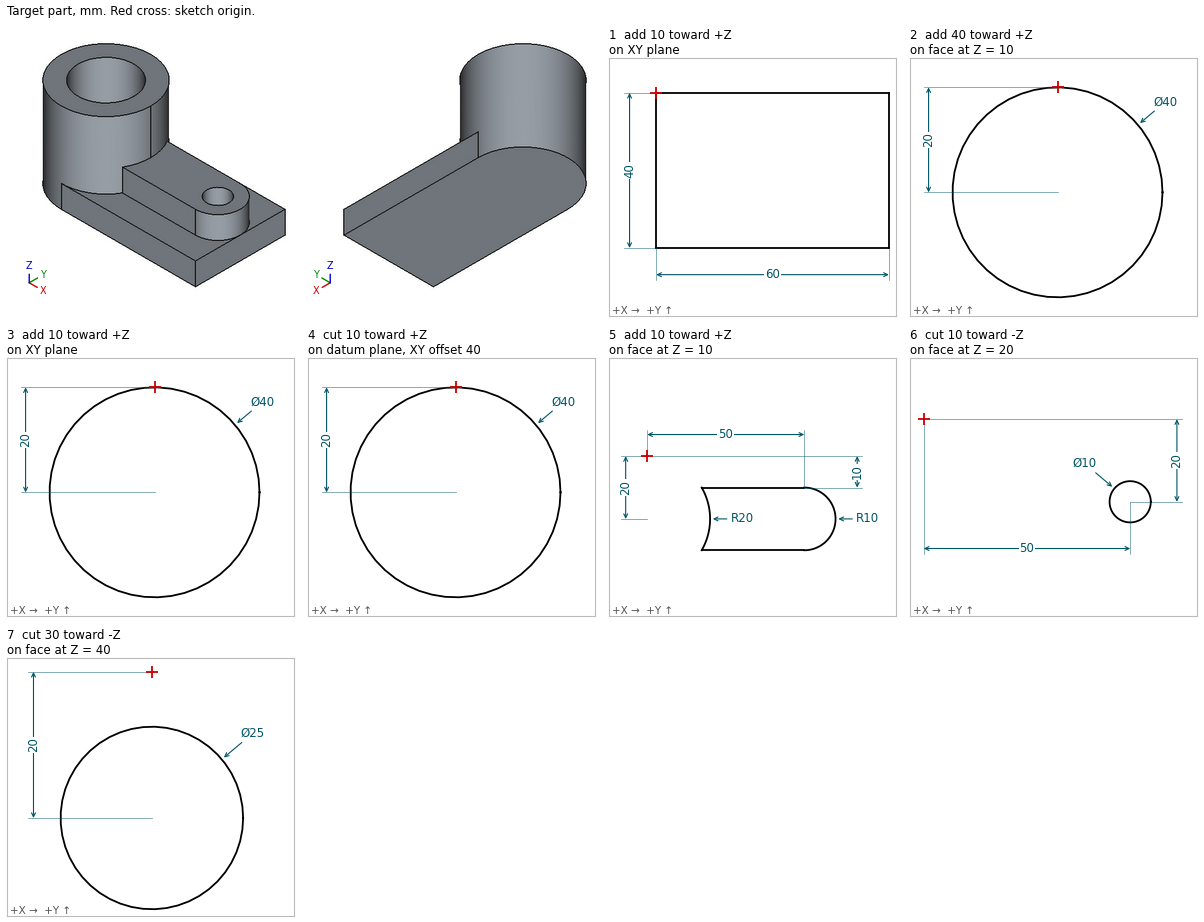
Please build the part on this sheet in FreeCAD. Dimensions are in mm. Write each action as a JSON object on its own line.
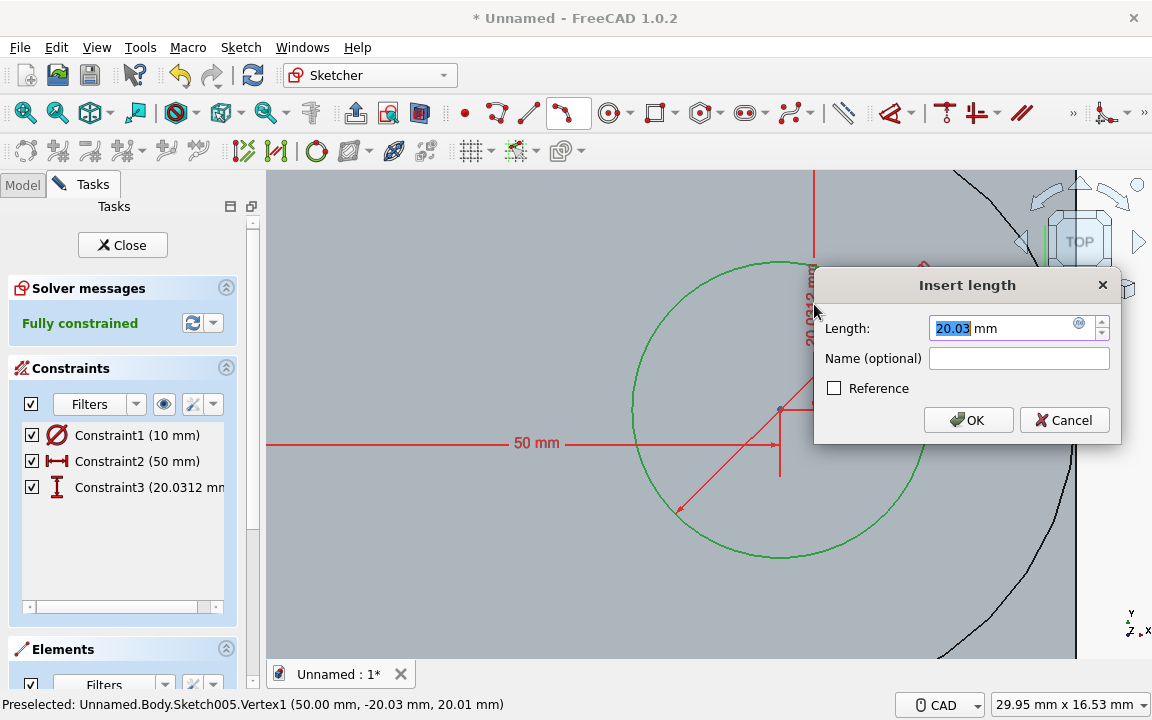
{"action": "type", "text": "20"}
{"action": "key", "text": "Return"}
{"action": "key", "text": "Escape"}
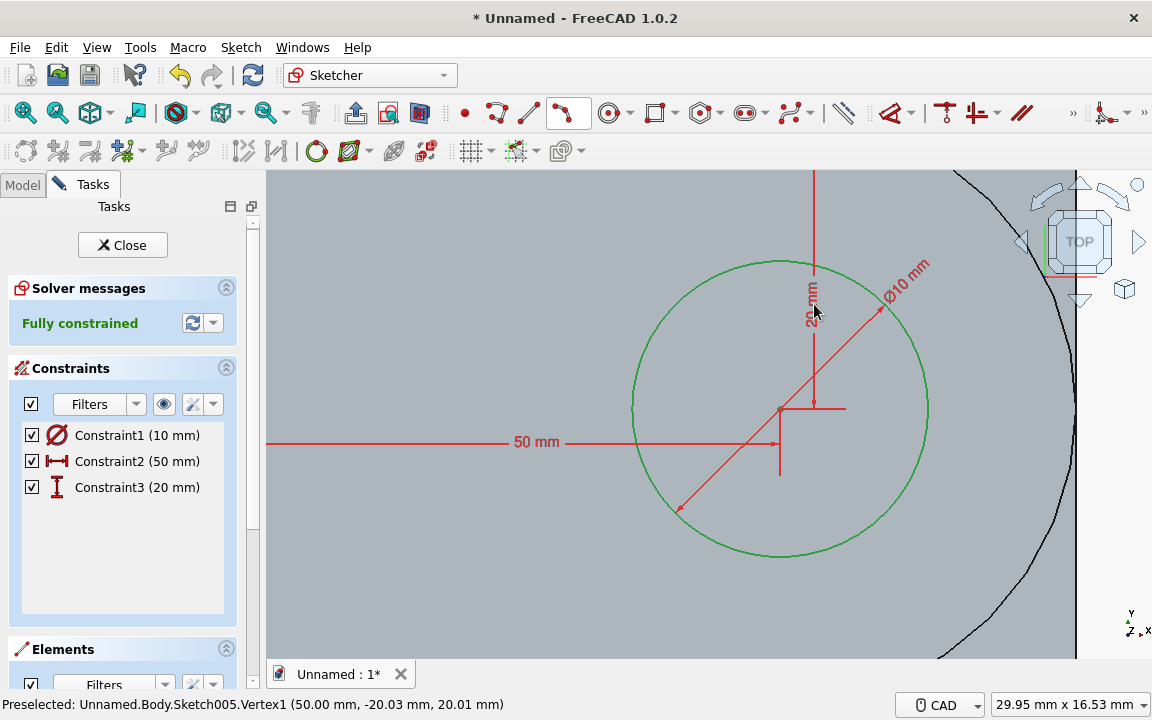
{"action": "left_click", "coordinate": [123, 245]}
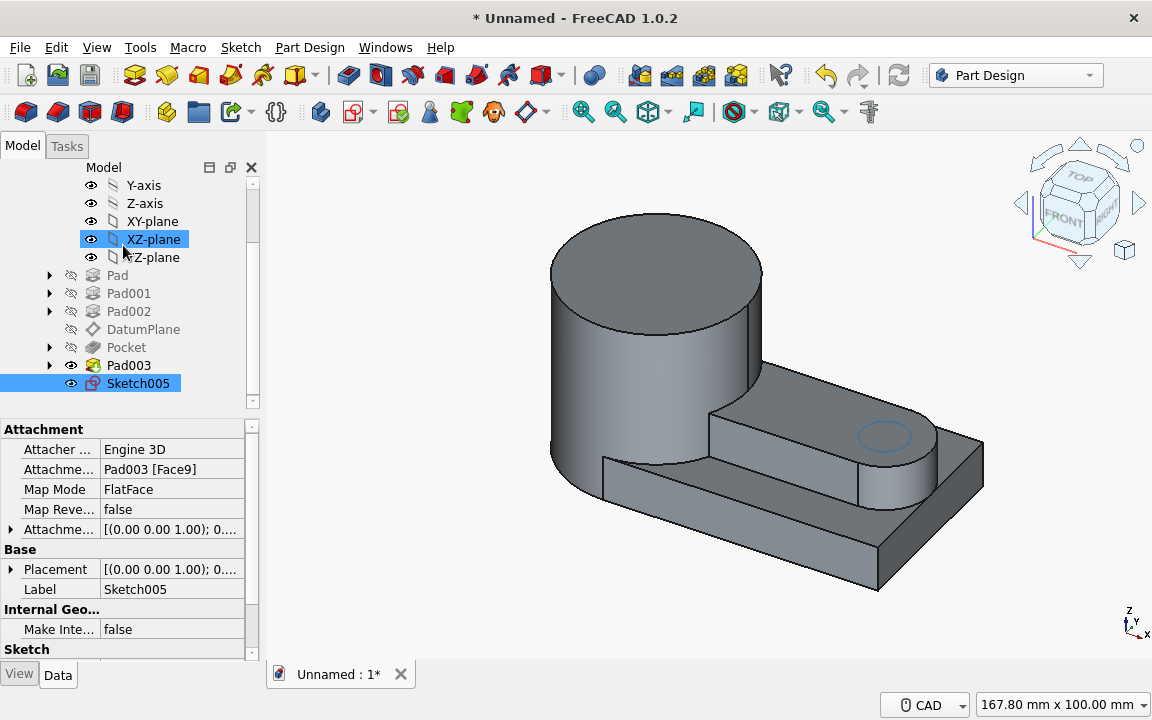
{"action": "left_click", "coordinate": [350, 76]}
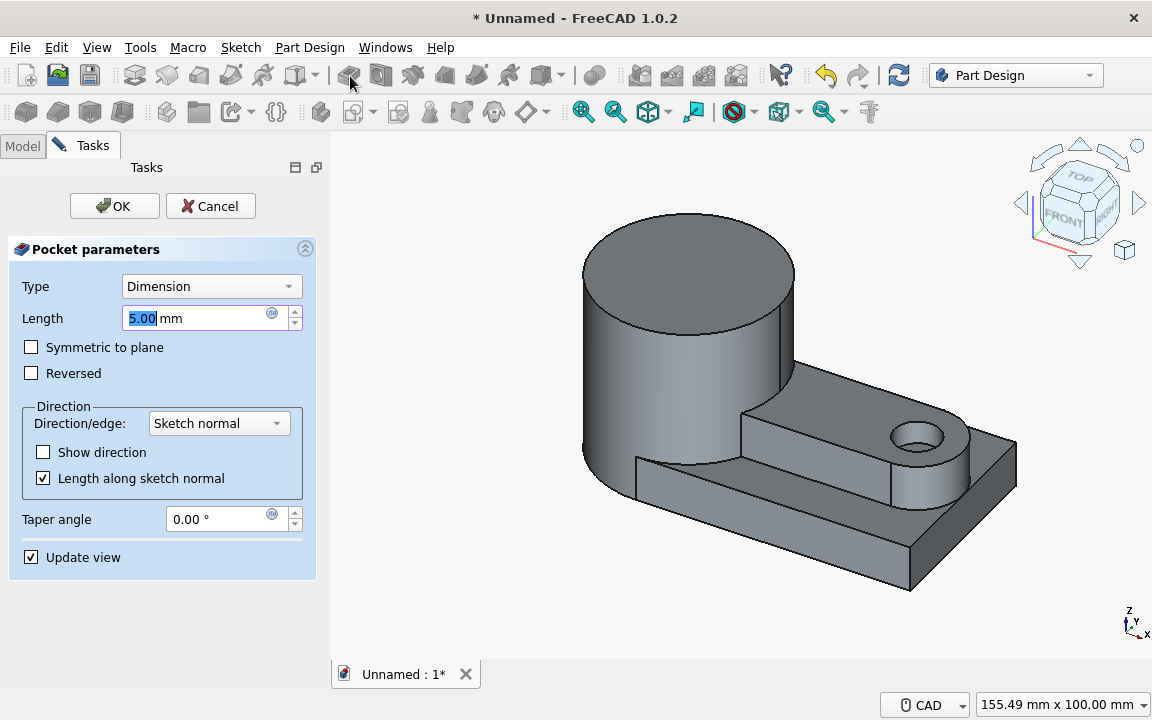
{"action": "type", "text": "10"}
{"action": "key", "text": "Tab"}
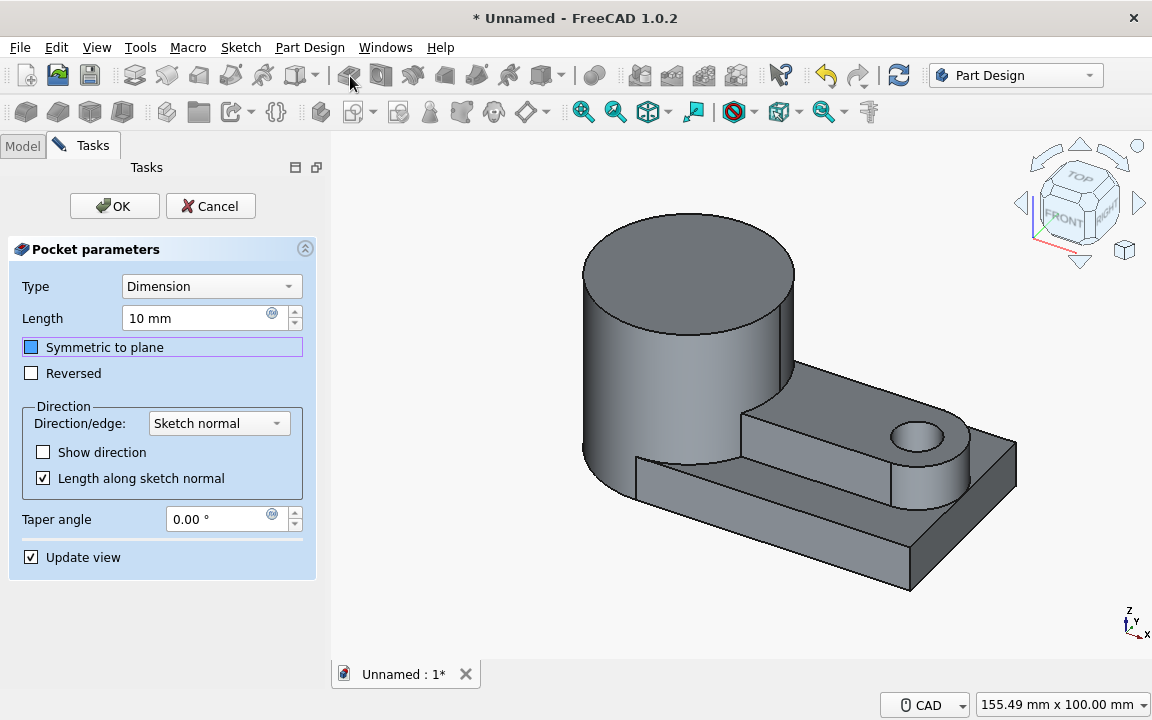
{"action": "left_click", "coordinate": [115, 206]}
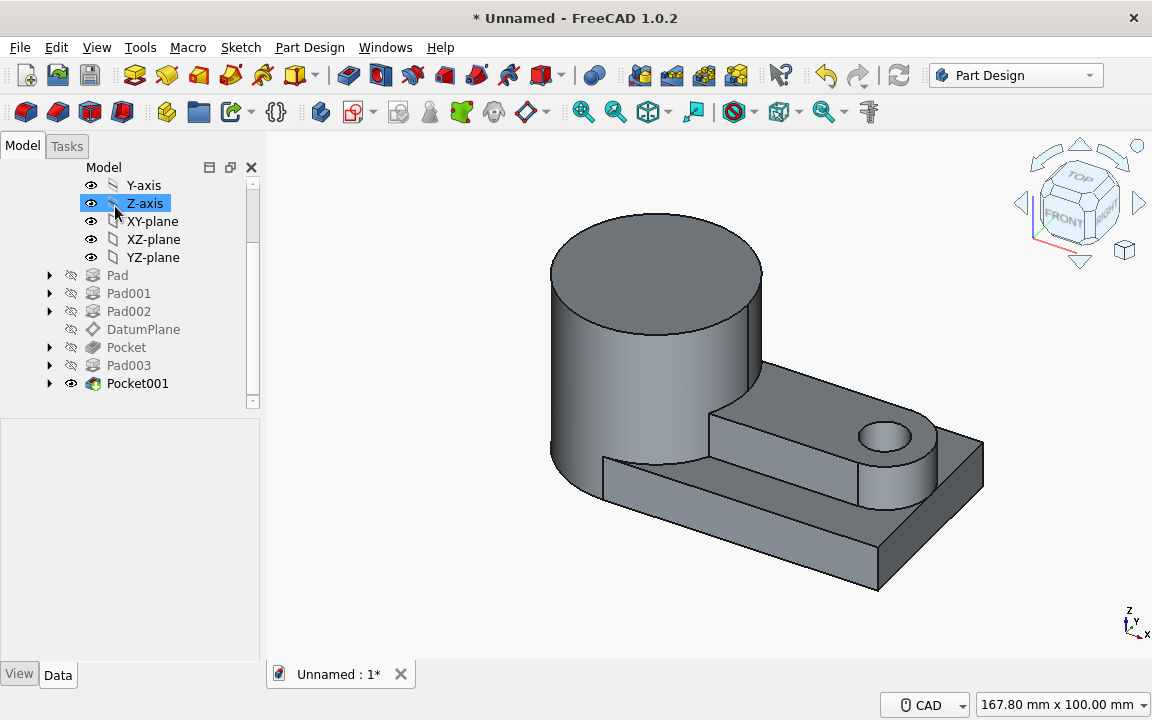
{"action": "left_click", "coordinate": [656, 273]}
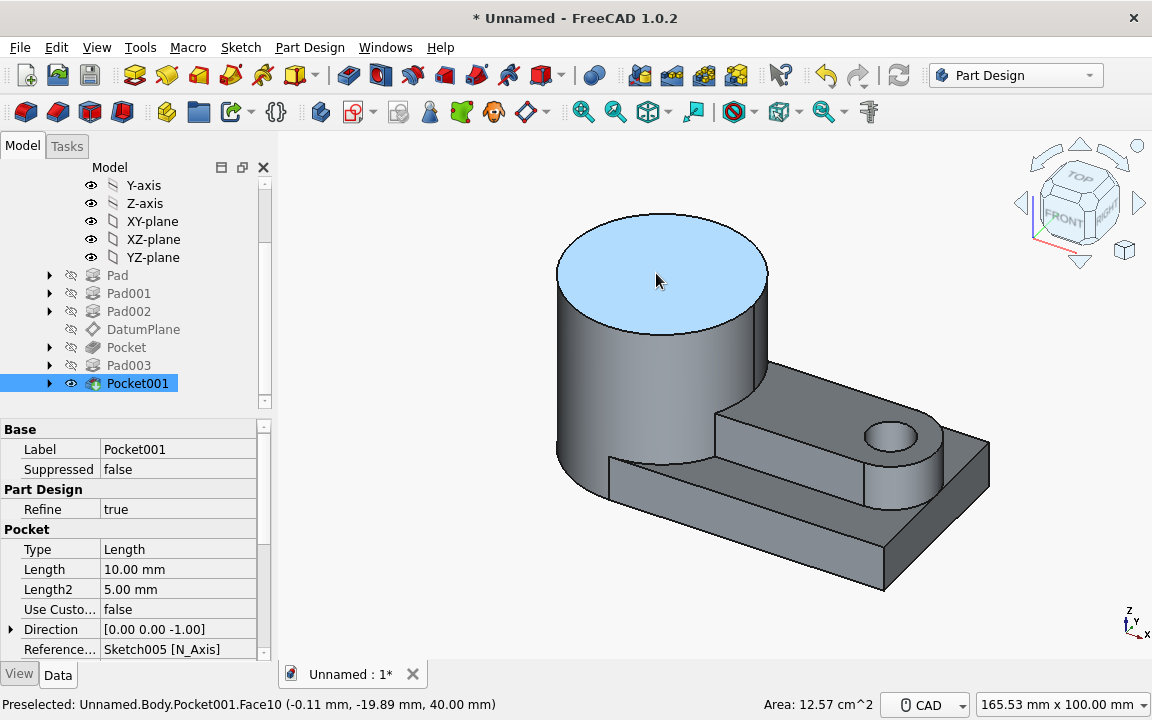
{"action": "left_click", "coordinate": [354, 112]}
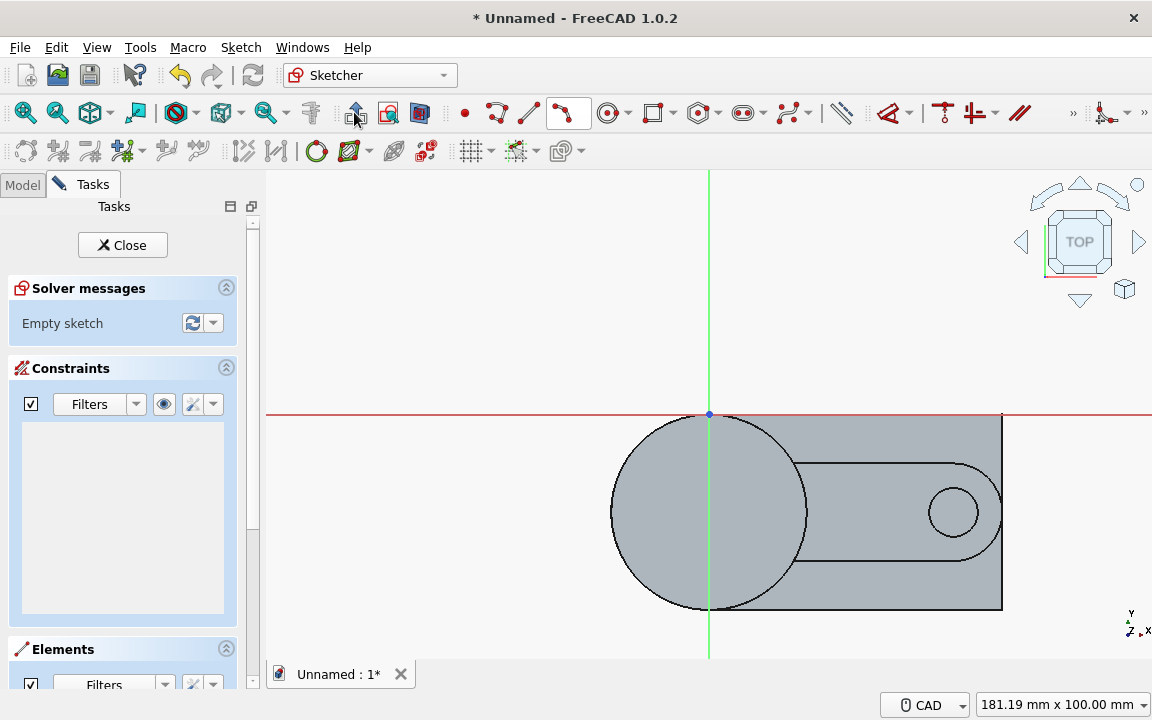
{"action": "scroll", "coordinate": [792, 591], "scroll_direction": "up", "scroll_amount": 3}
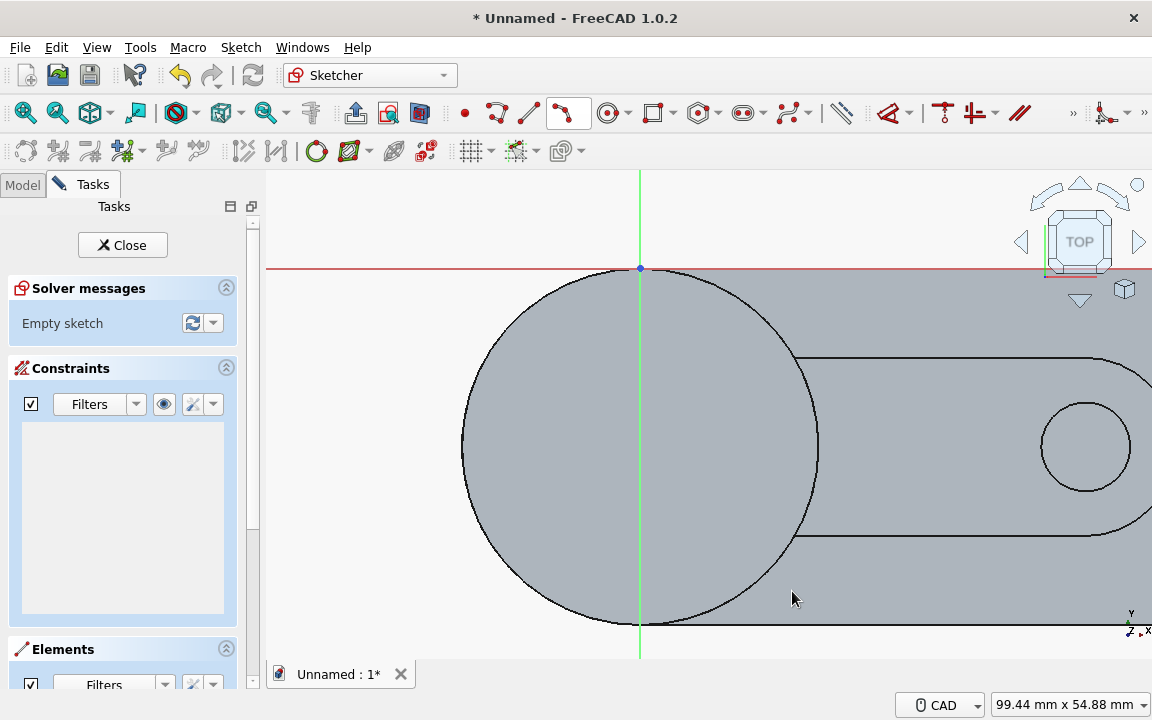
{"action": "left_click", "coordinate": [608, 114]}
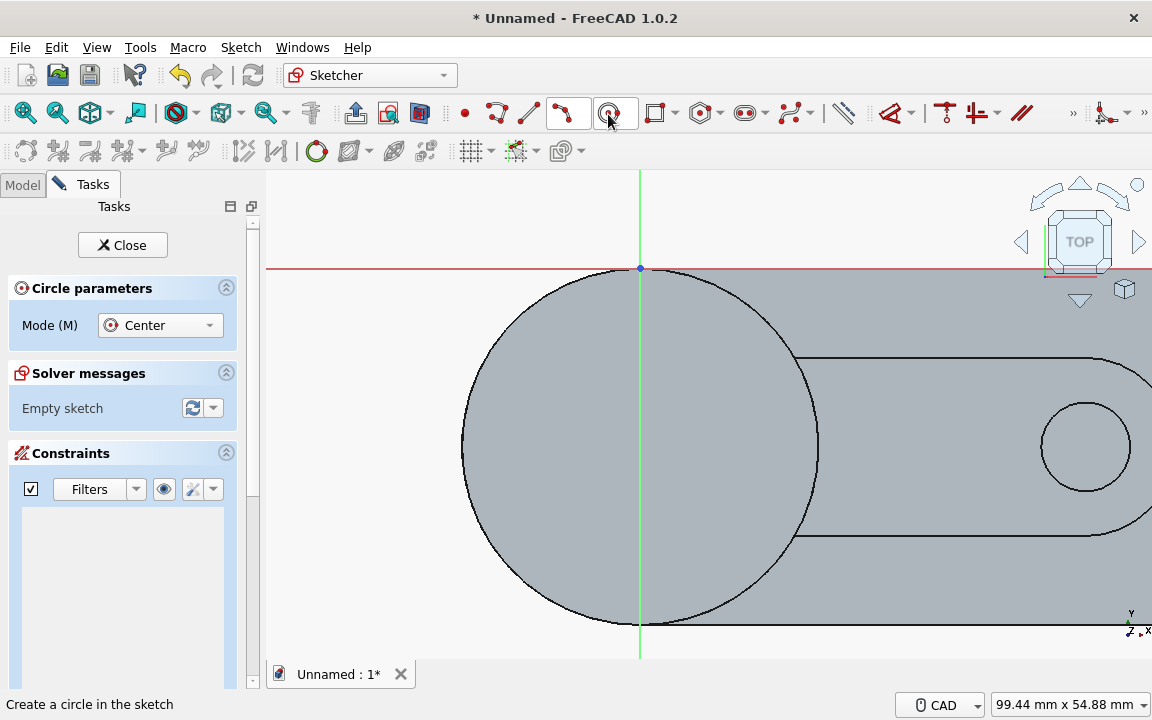
{"action": "left_click", "coordinate": [640, 447]}
{"action": "left_click", "coordinate": [719, 368]}
{"action": "key", "text": "Escape"}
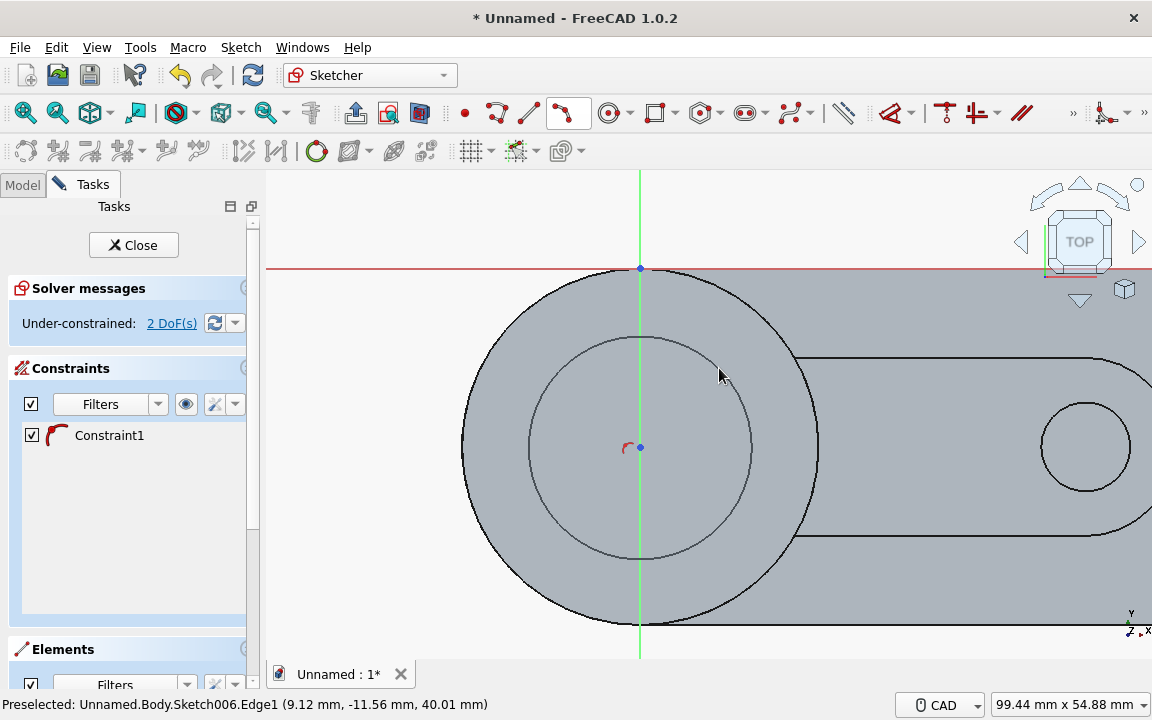
{"action": "left_click", "coordinate": [890, 114]}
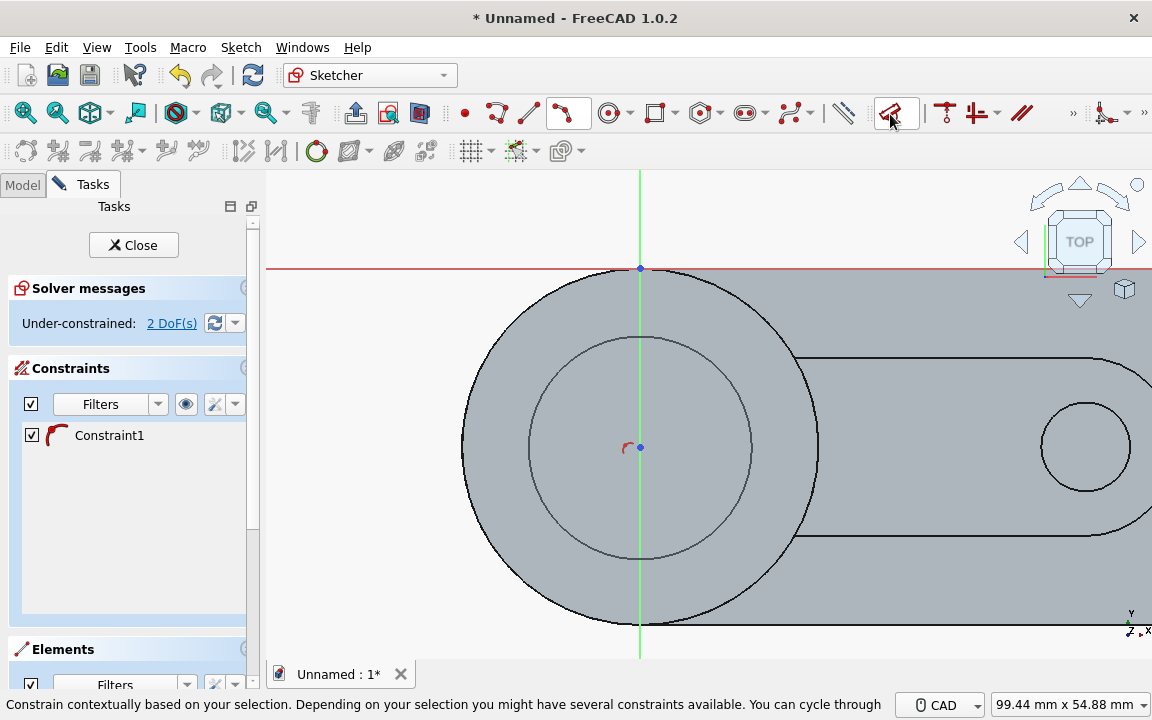
{"action": "left_click", "coordinate": [719, 369]}
{"action": "left_click", "coordinate": [742, 346]}